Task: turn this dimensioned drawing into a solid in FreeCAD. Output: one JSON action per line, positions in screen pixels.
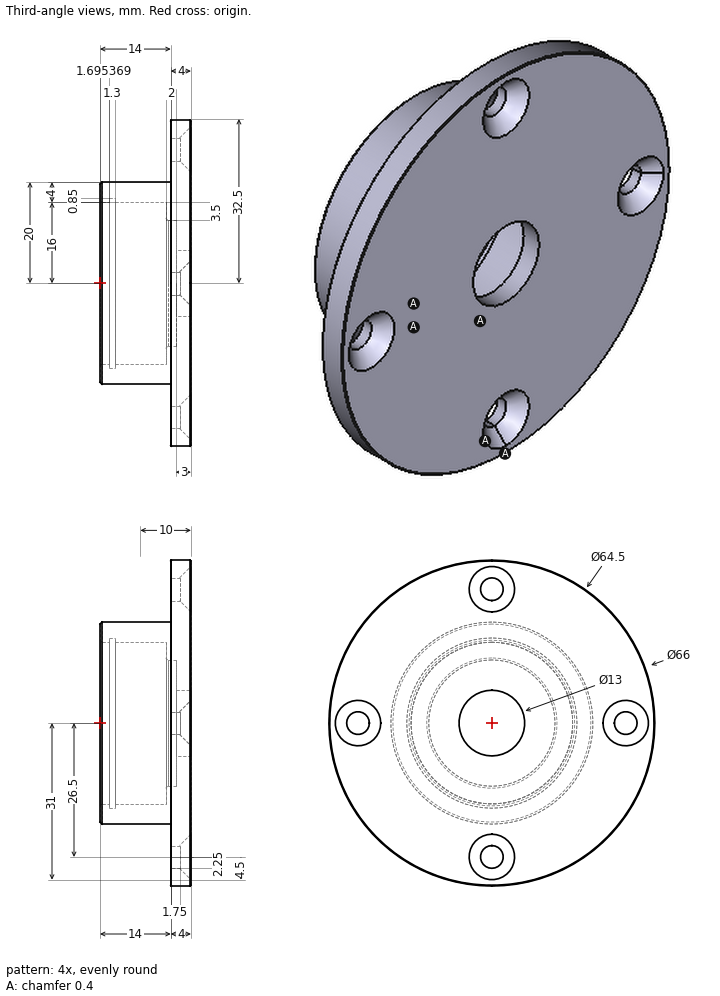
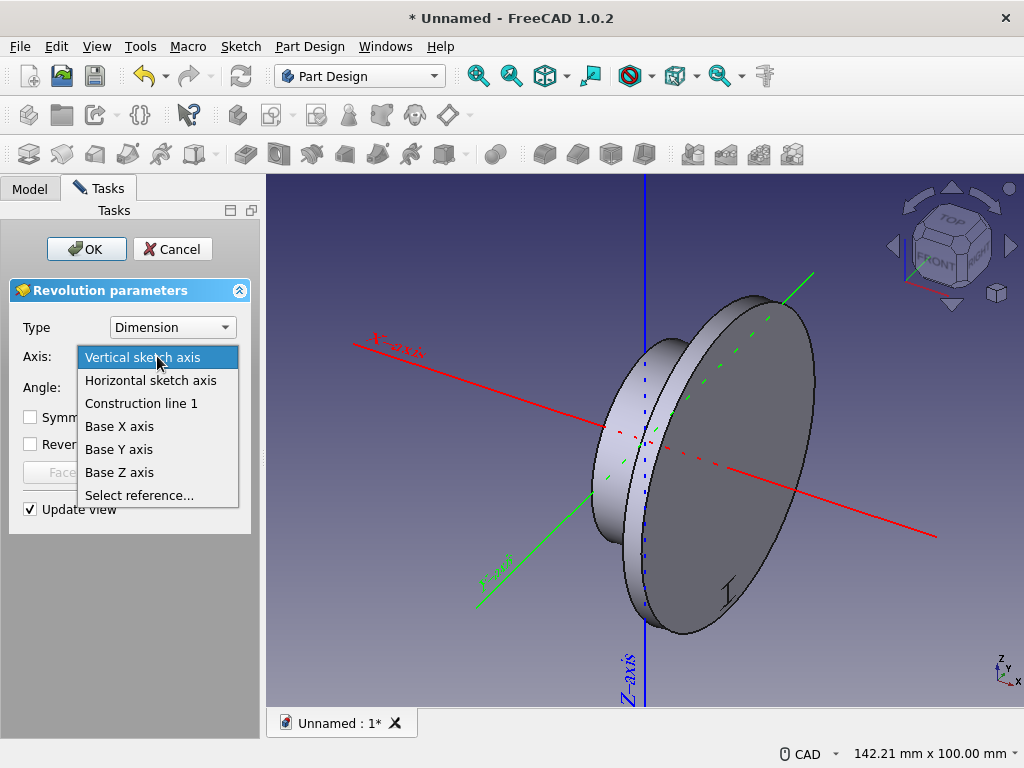
{"action": "left_click", "coordinate": [156, 404]}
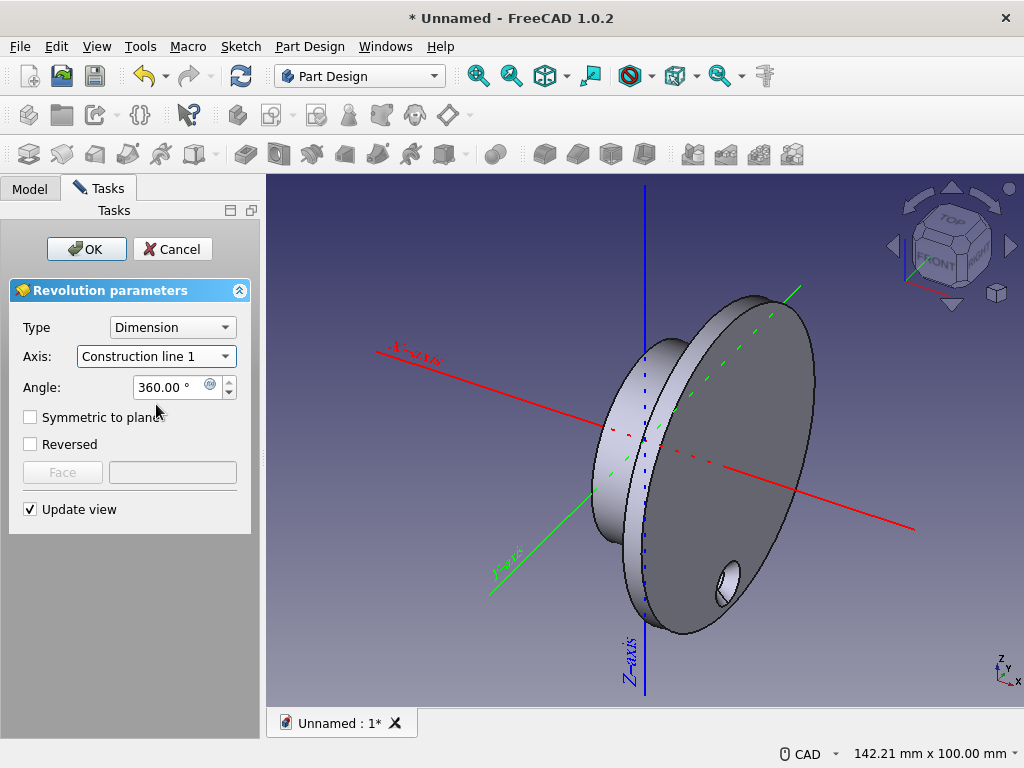
{"action": "left_click", "coordinate": [87, 249]}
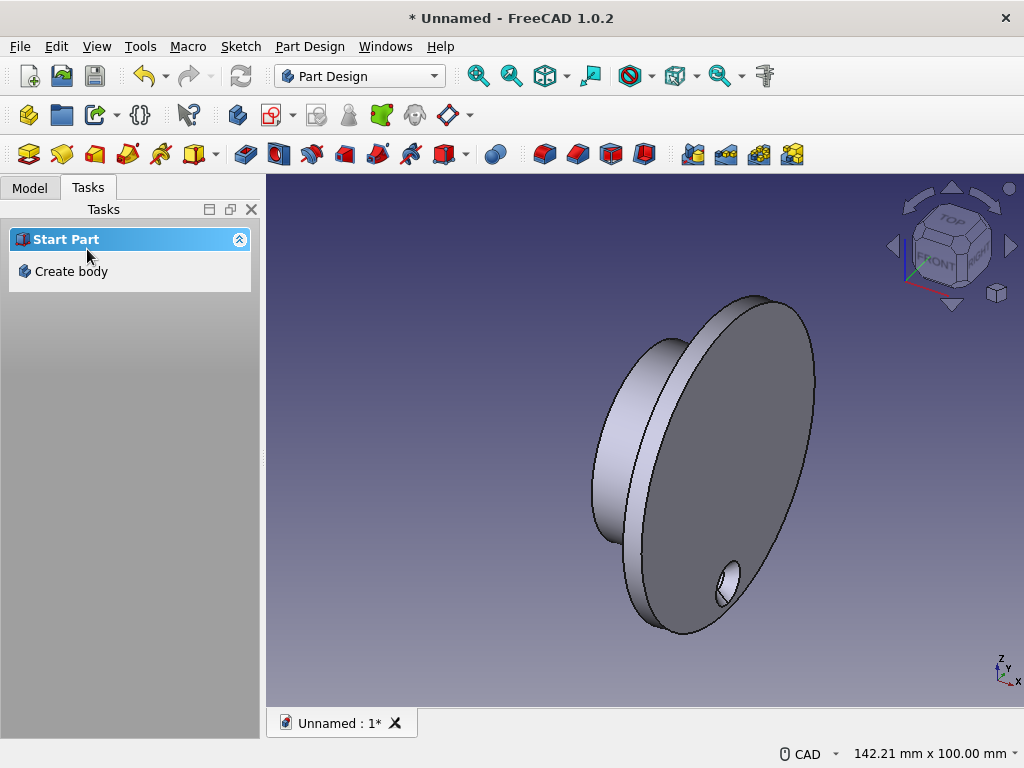
{"action": "left_click", "coordinate": [30, 188]}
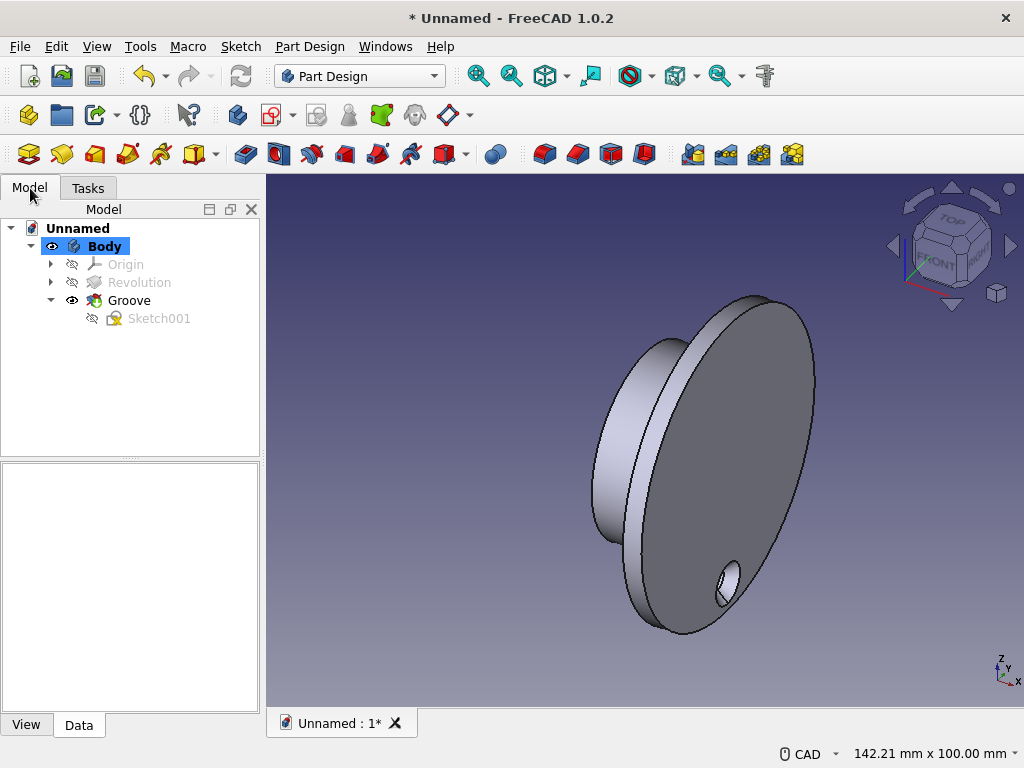
{"action": "left_click", "coordinate": [117, 300]}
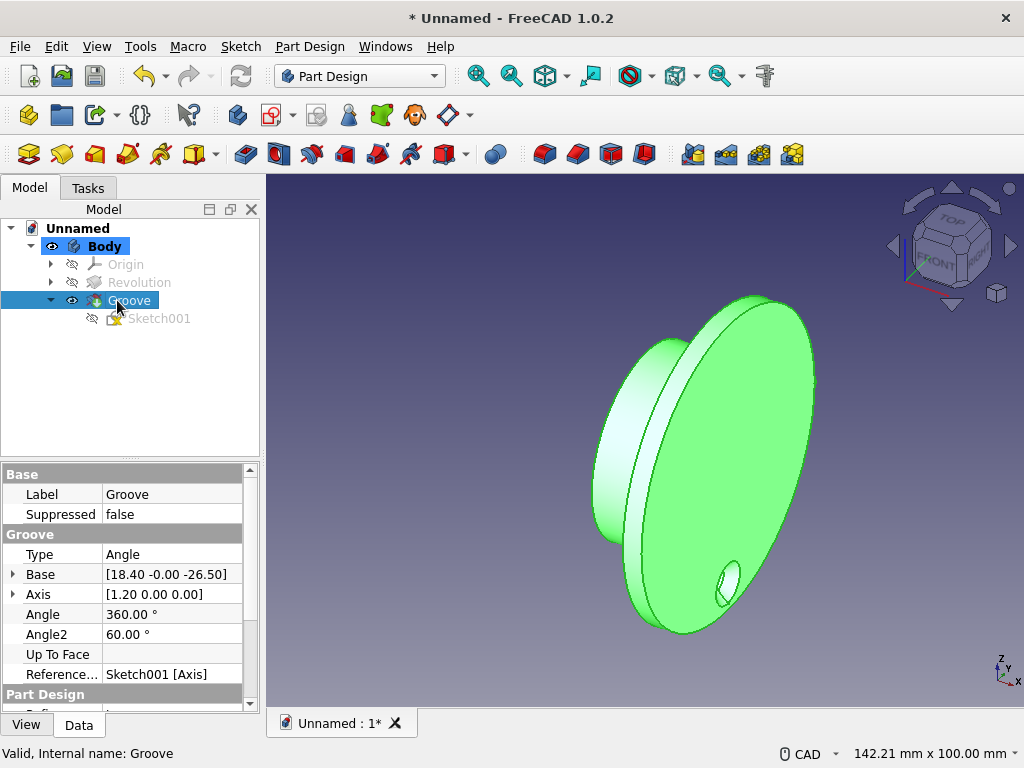
{"action": "left_click", "coordinate": [759, 154]}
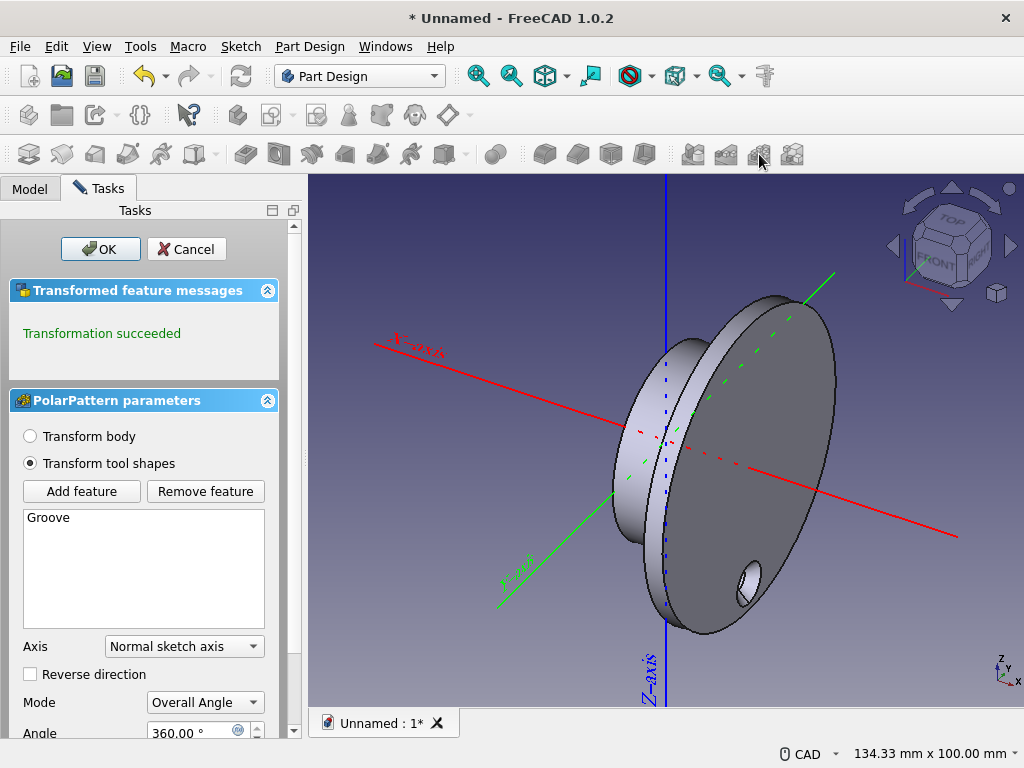
{"action": "left_click", "coordinate": [185, 646]}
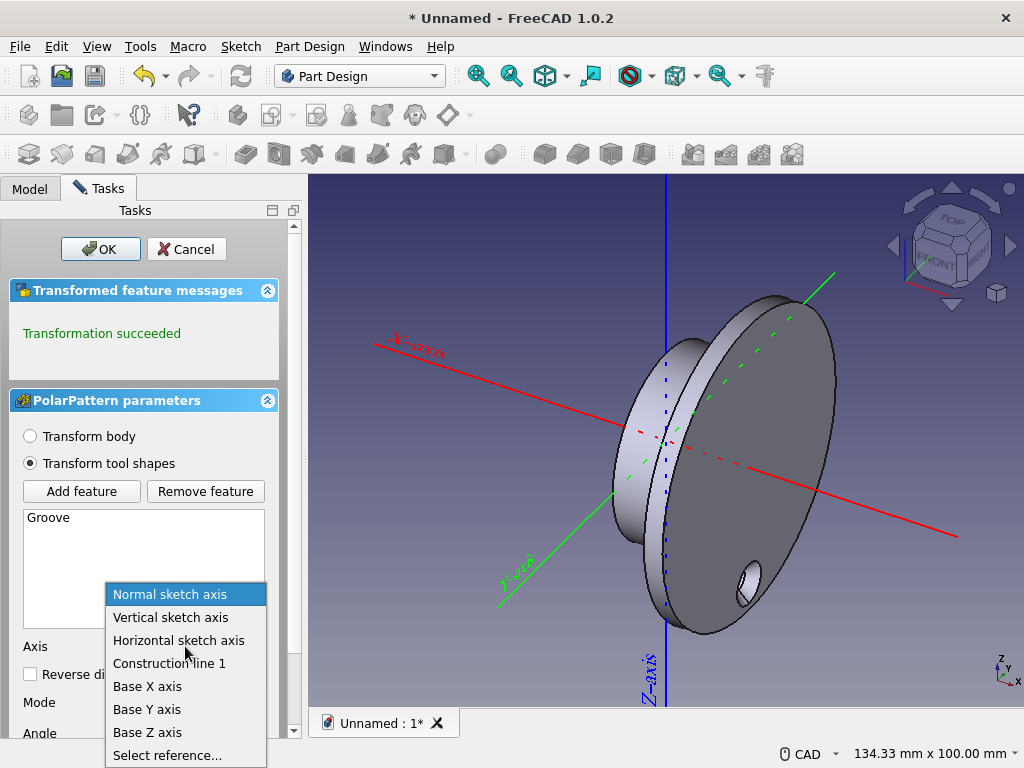
{"action": "left_click", "coordinate": [184, 686]}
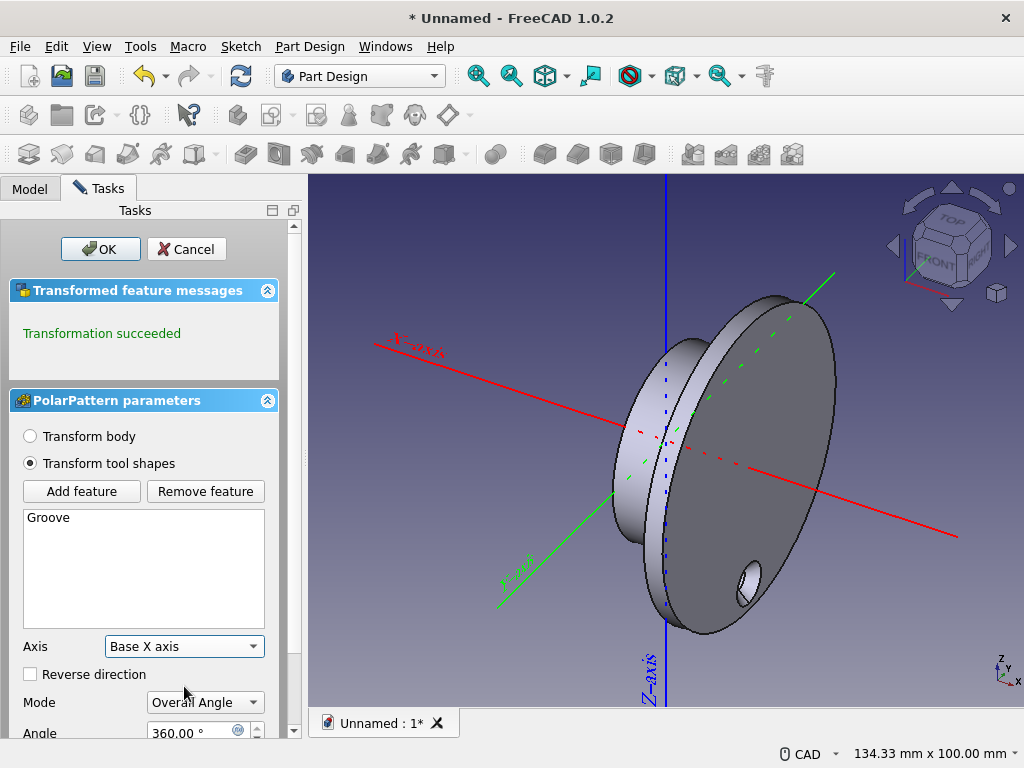
{"action": "scroll", "coordinate": [294, 479], "scroll_direction": "down", "scroll_amount": 2}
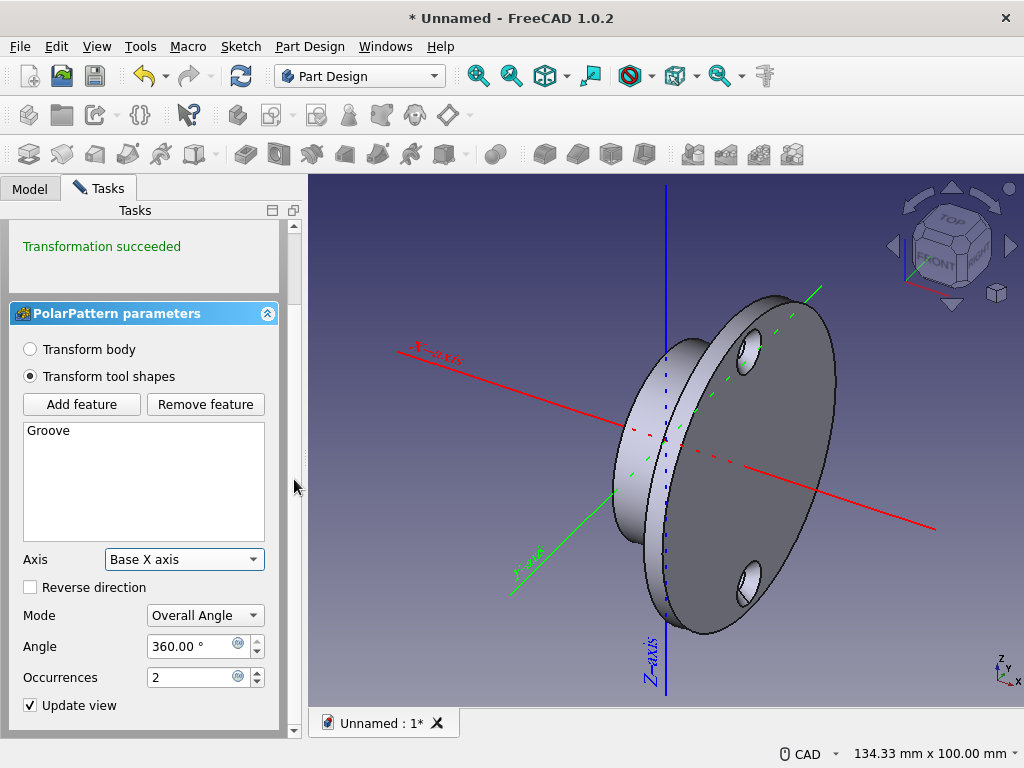
{"action": "triple_click", "coordinate": [199, 678]}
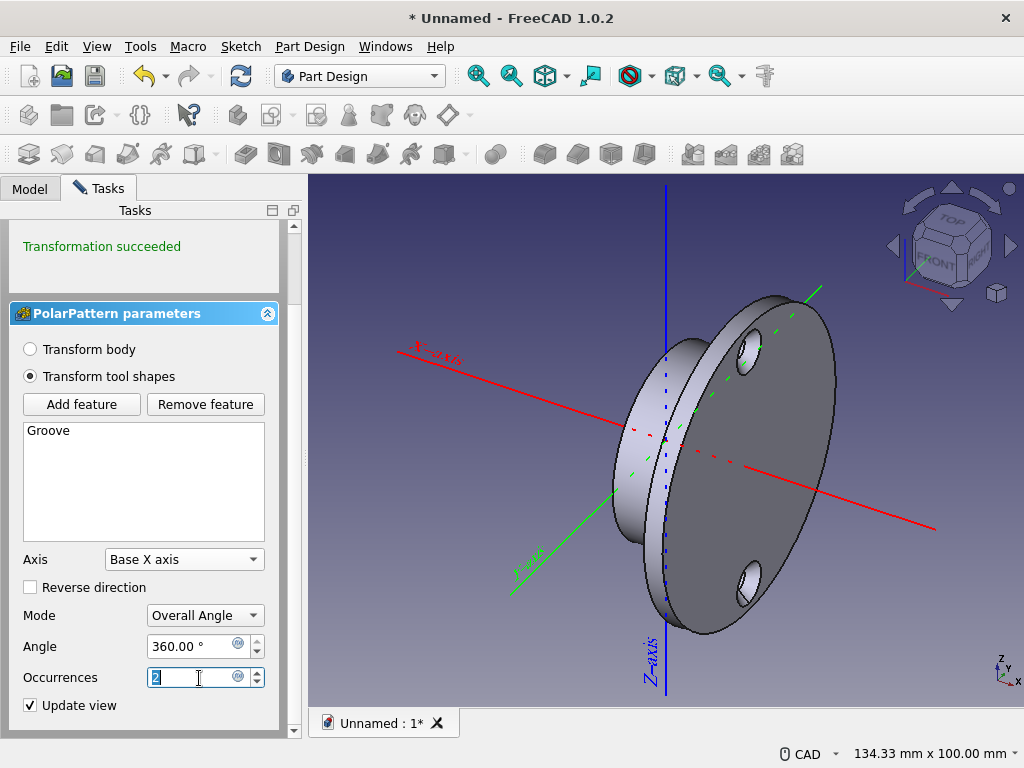
{"action": "type", "text": "4"}
{"action": "key", "text": "Tab"}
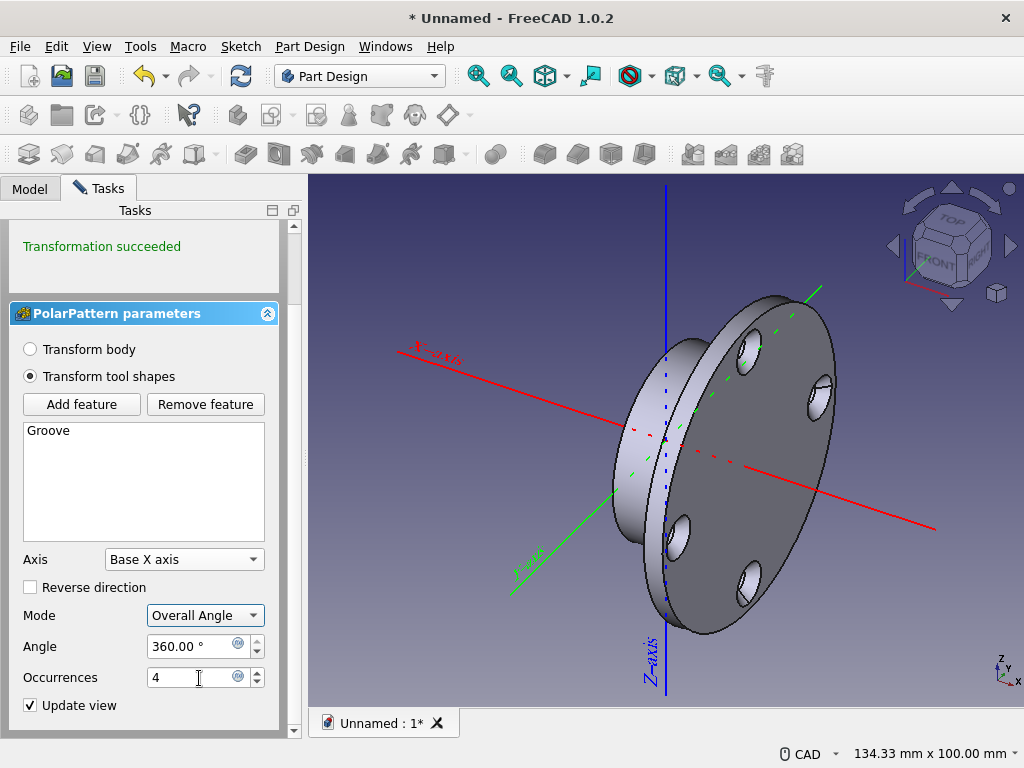
{"action": "scroll", "coordinate": [294, 479], "scroll_direction": "up", "scroll_amount": 3}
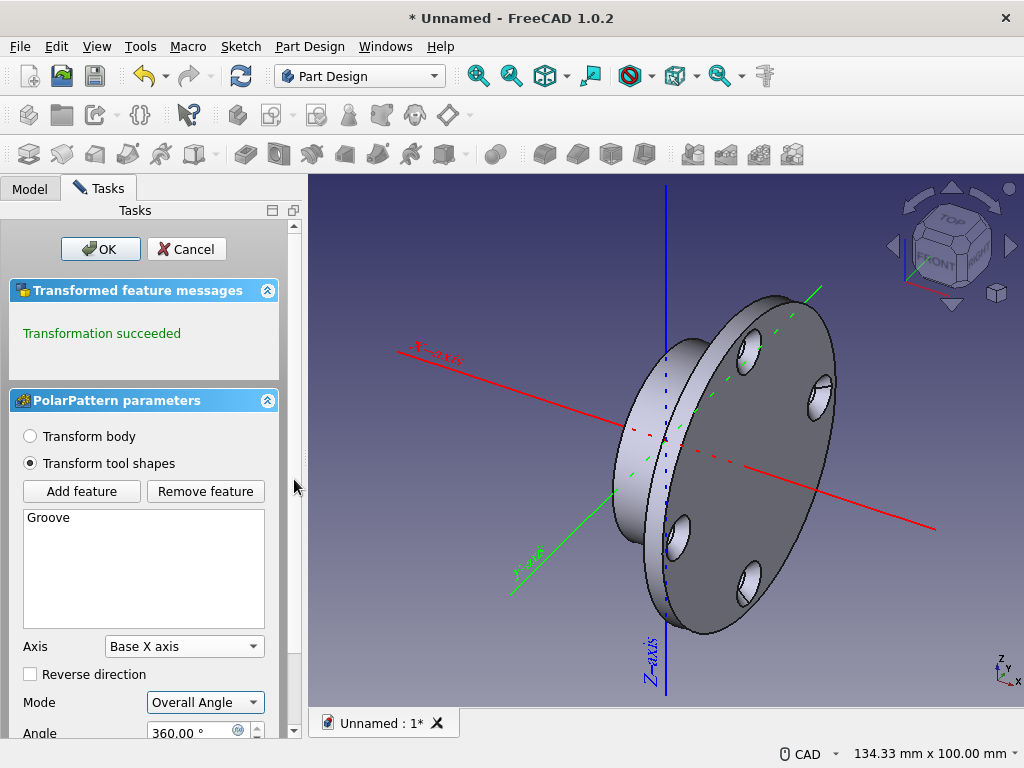
{"action": "left_click", "coordinate": [101, 249]}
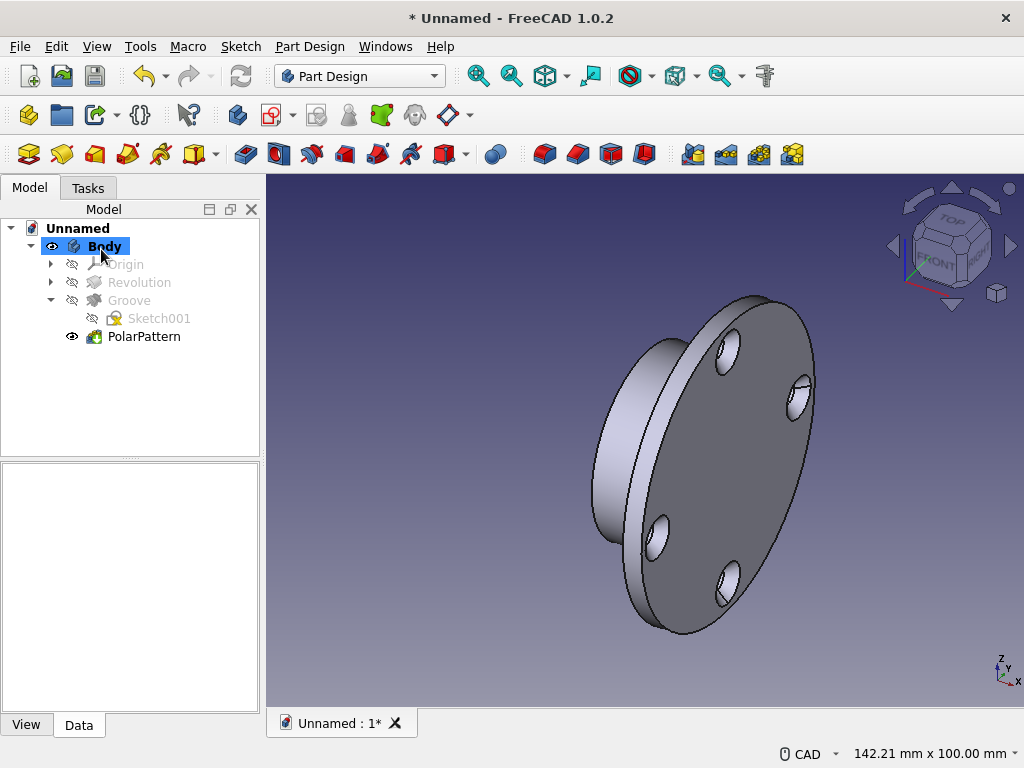
{"action": "left_click", "coordinate": [641, 553]}